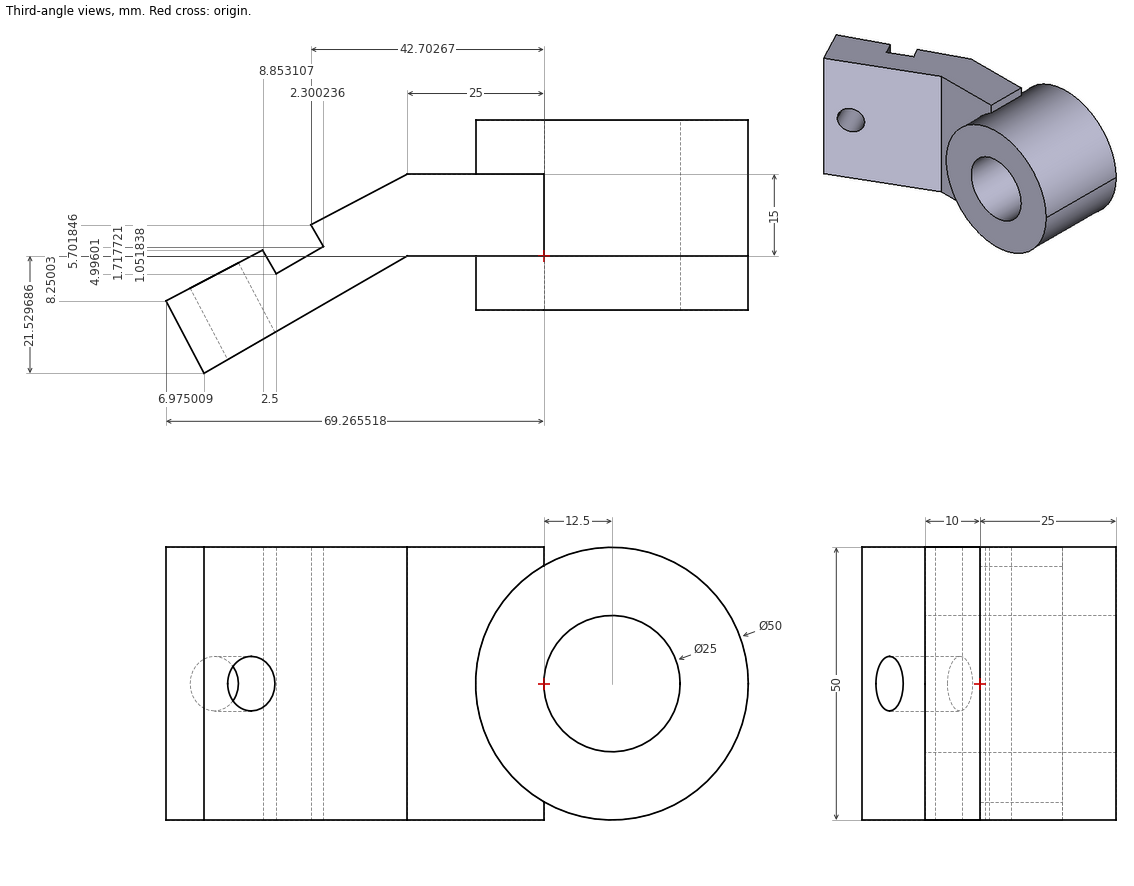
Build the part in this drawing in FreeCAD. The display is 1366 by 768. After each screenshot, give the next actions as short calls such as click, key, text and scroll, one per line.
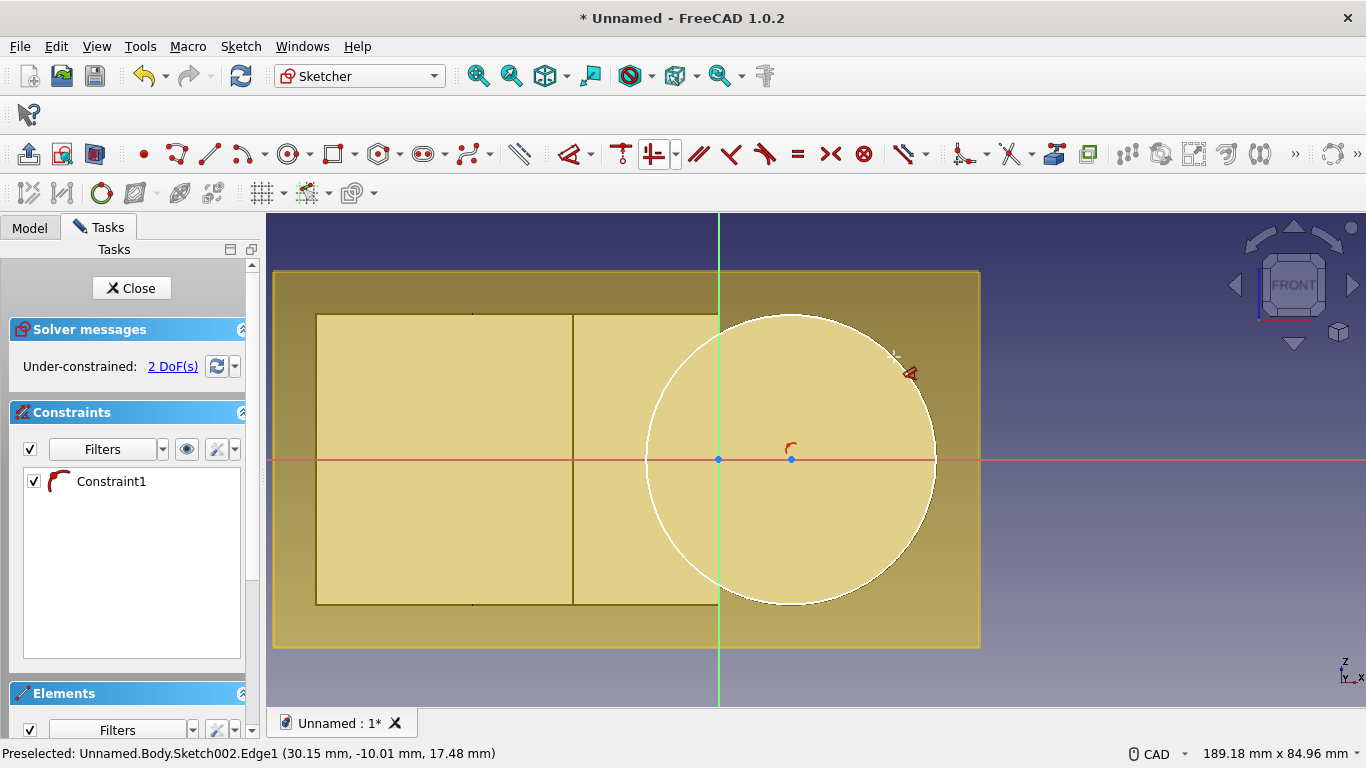
click(893, 357)
click(916, 334)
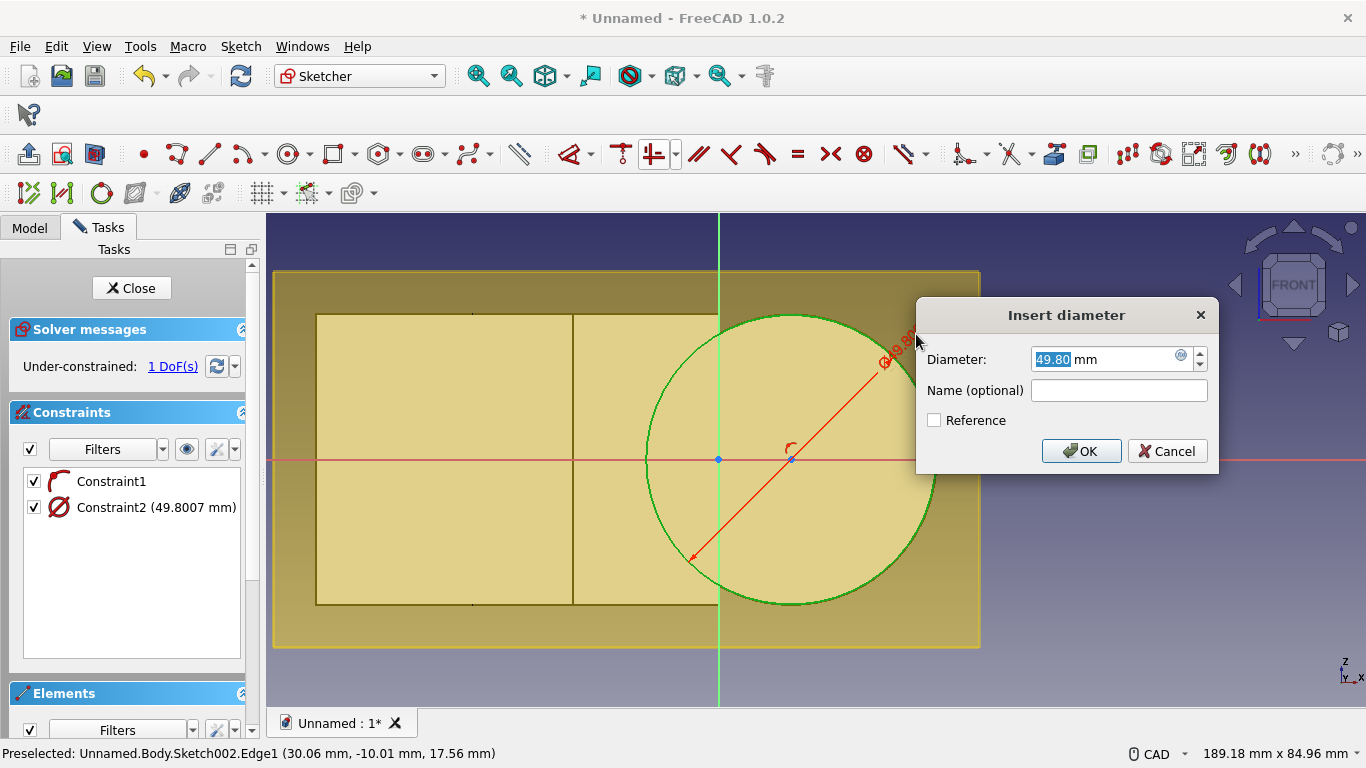
text(50)
key(Return)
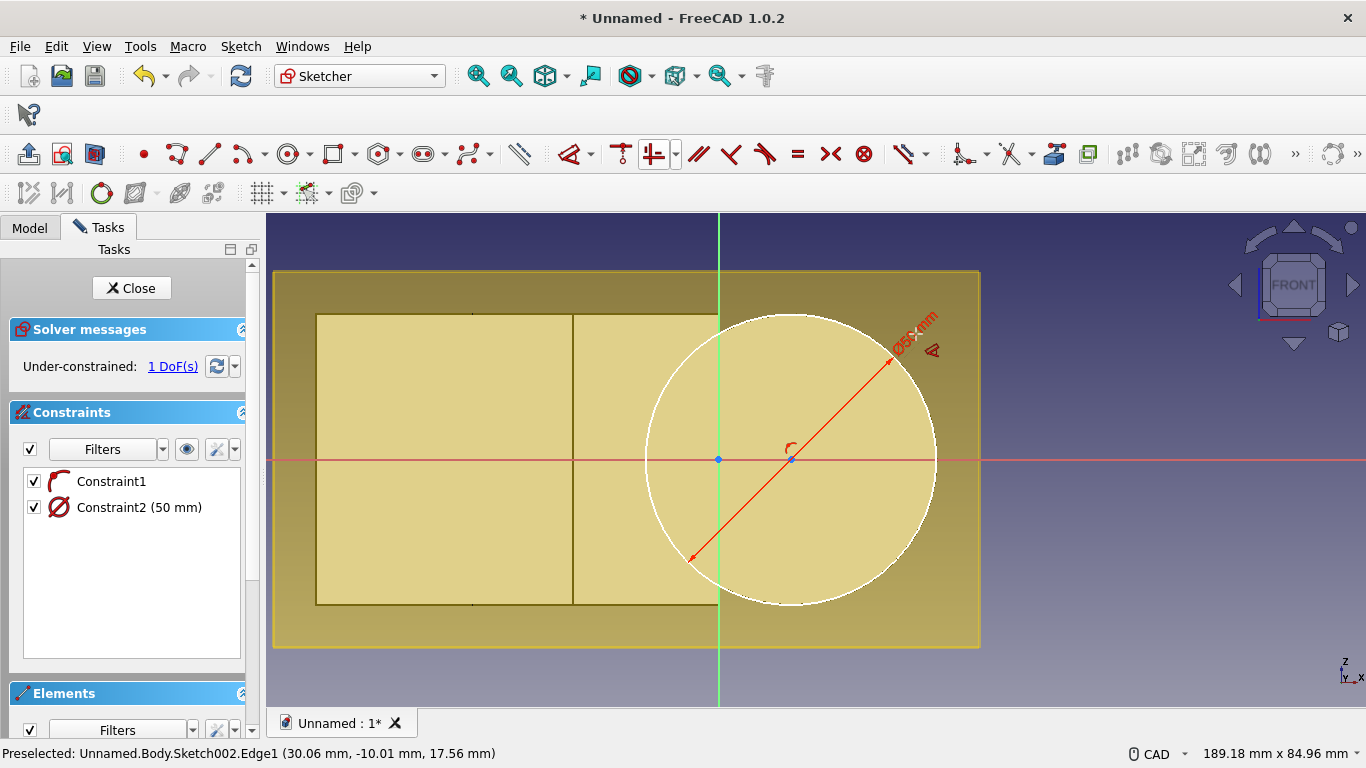
click(791, 460)
click(755, 494)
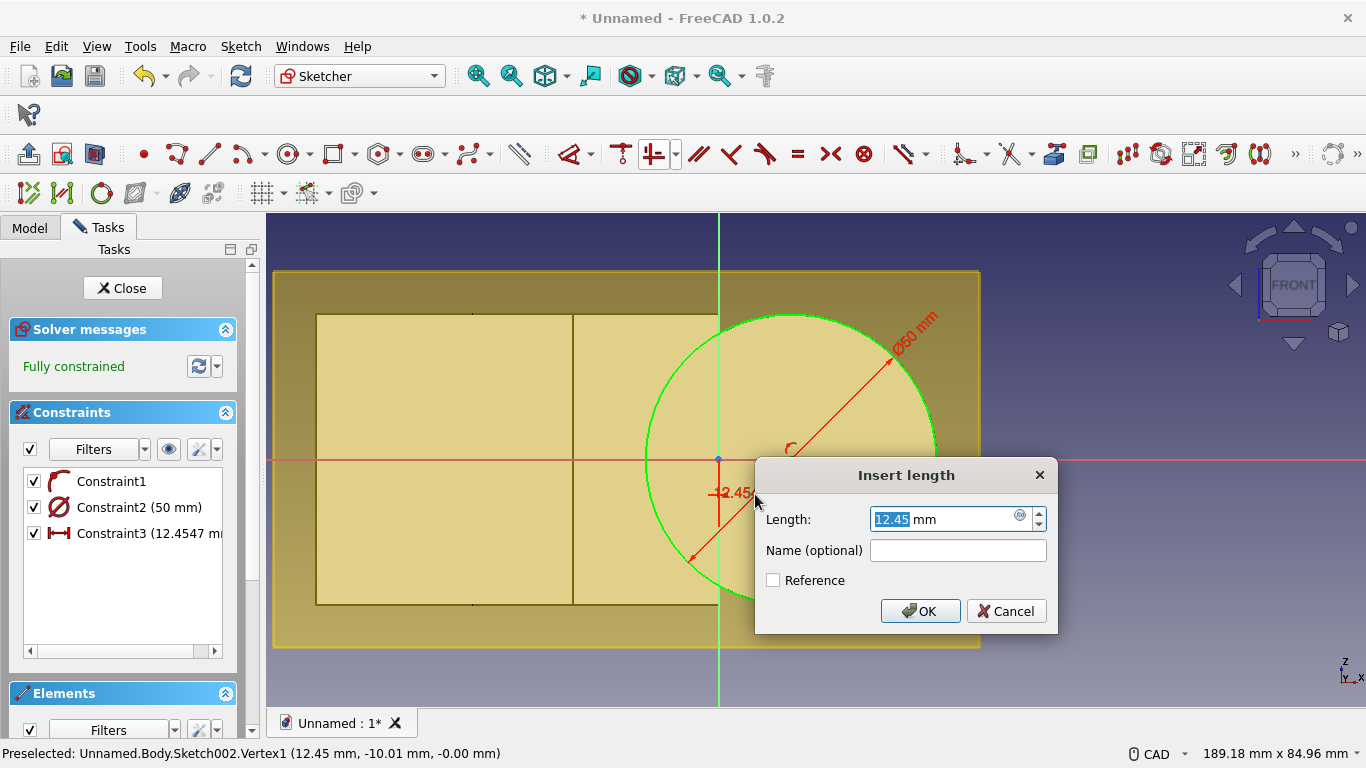
text(12.5)
key(Return)
key(Escape)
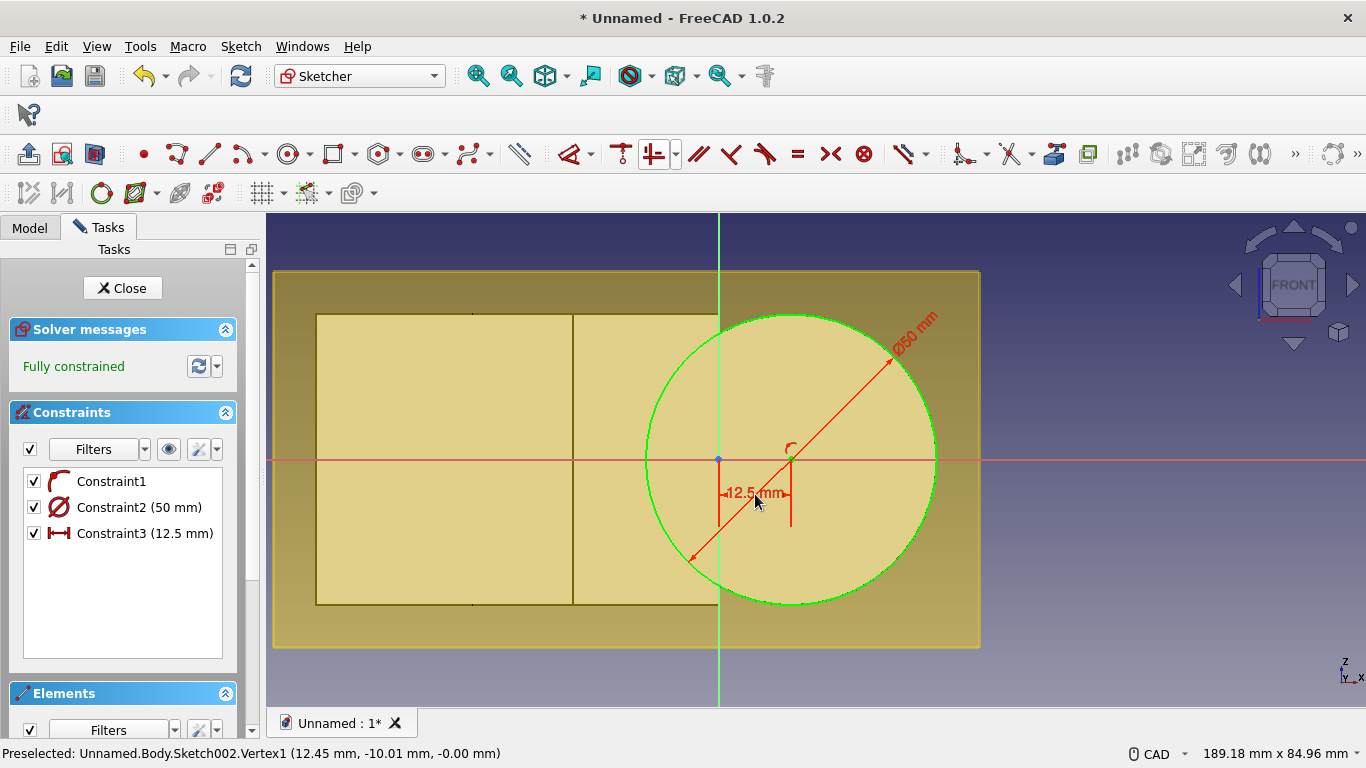
click(123, 288)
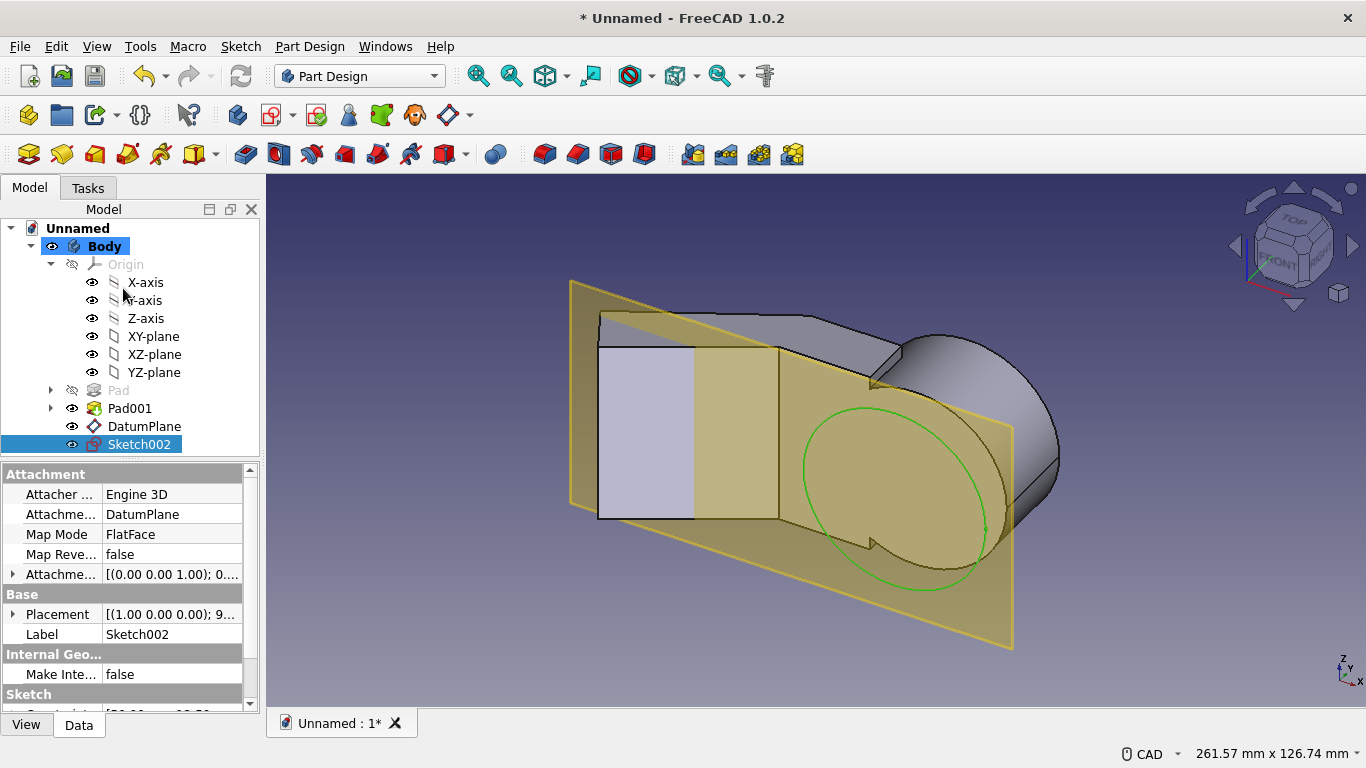
click(29, 154)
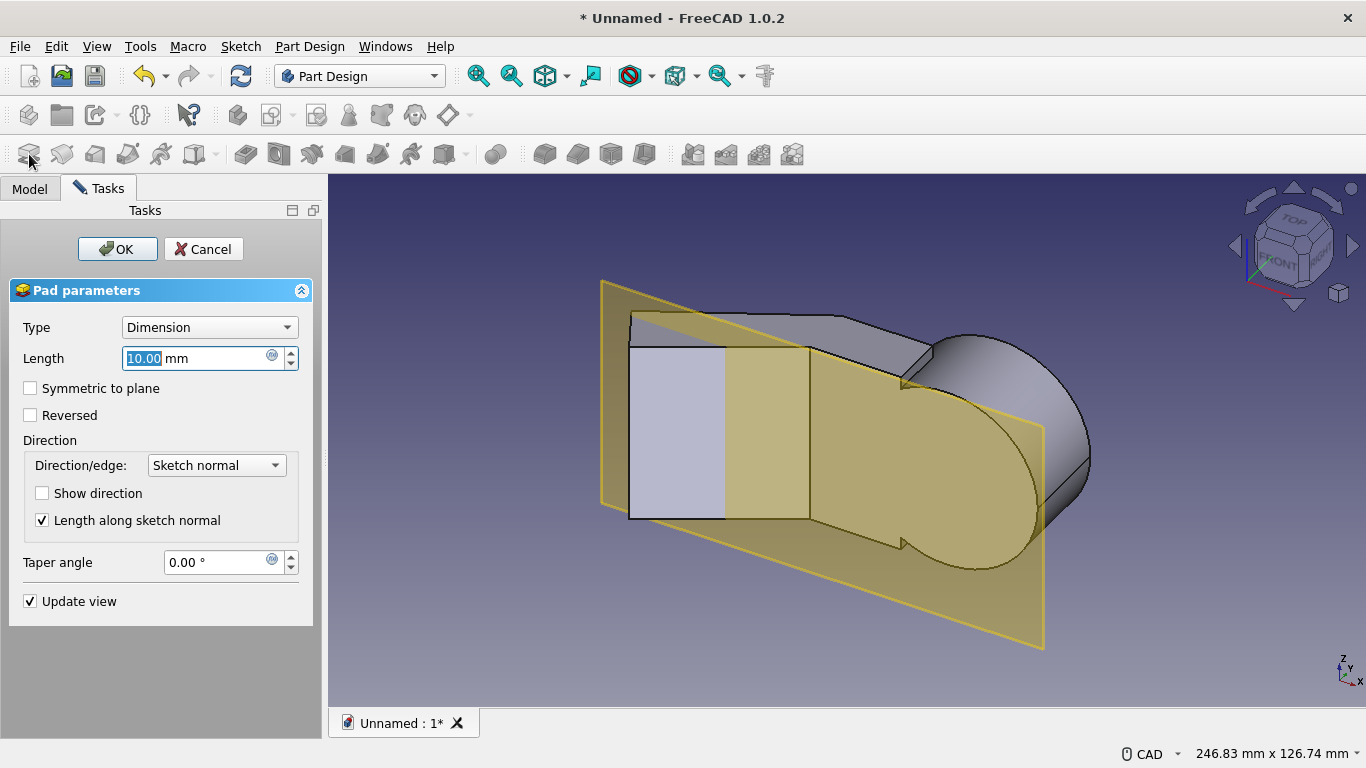
text(10)
key(Tab)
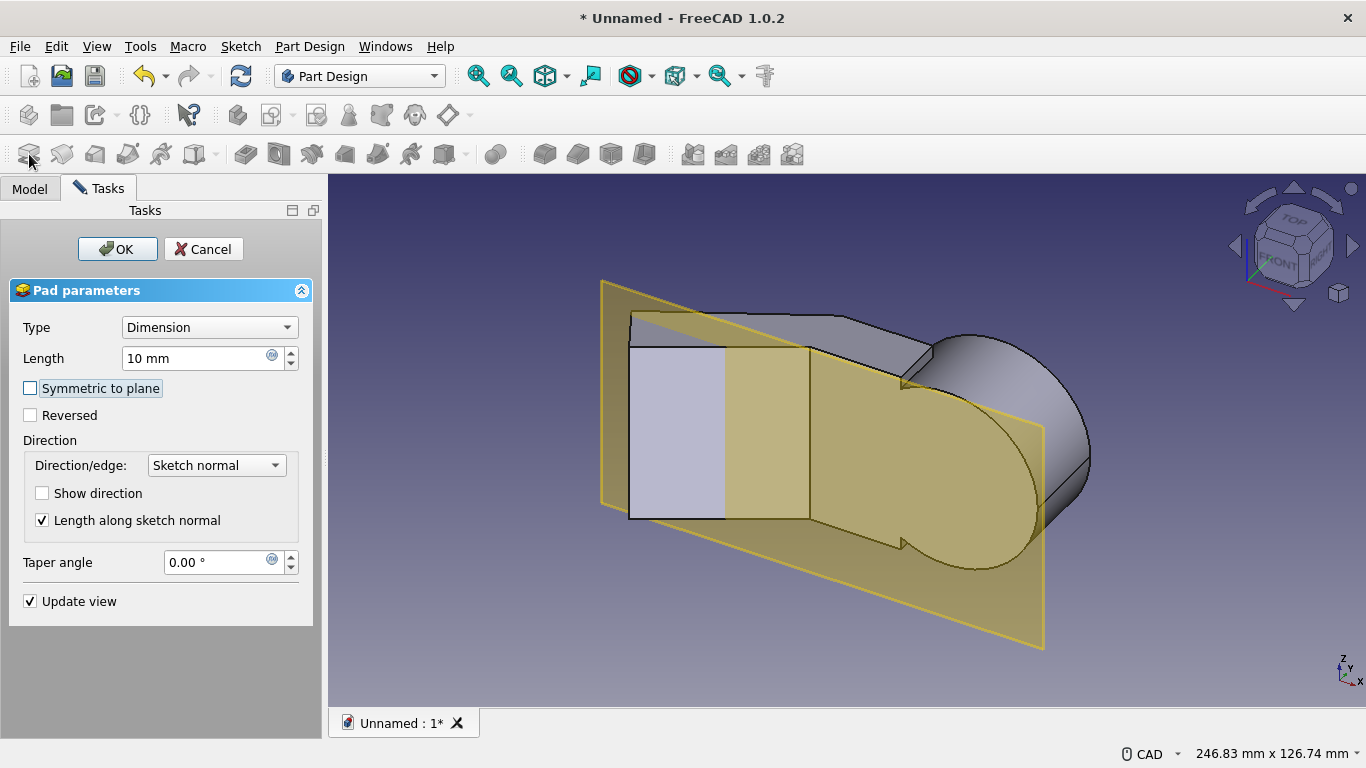
click(31, 415)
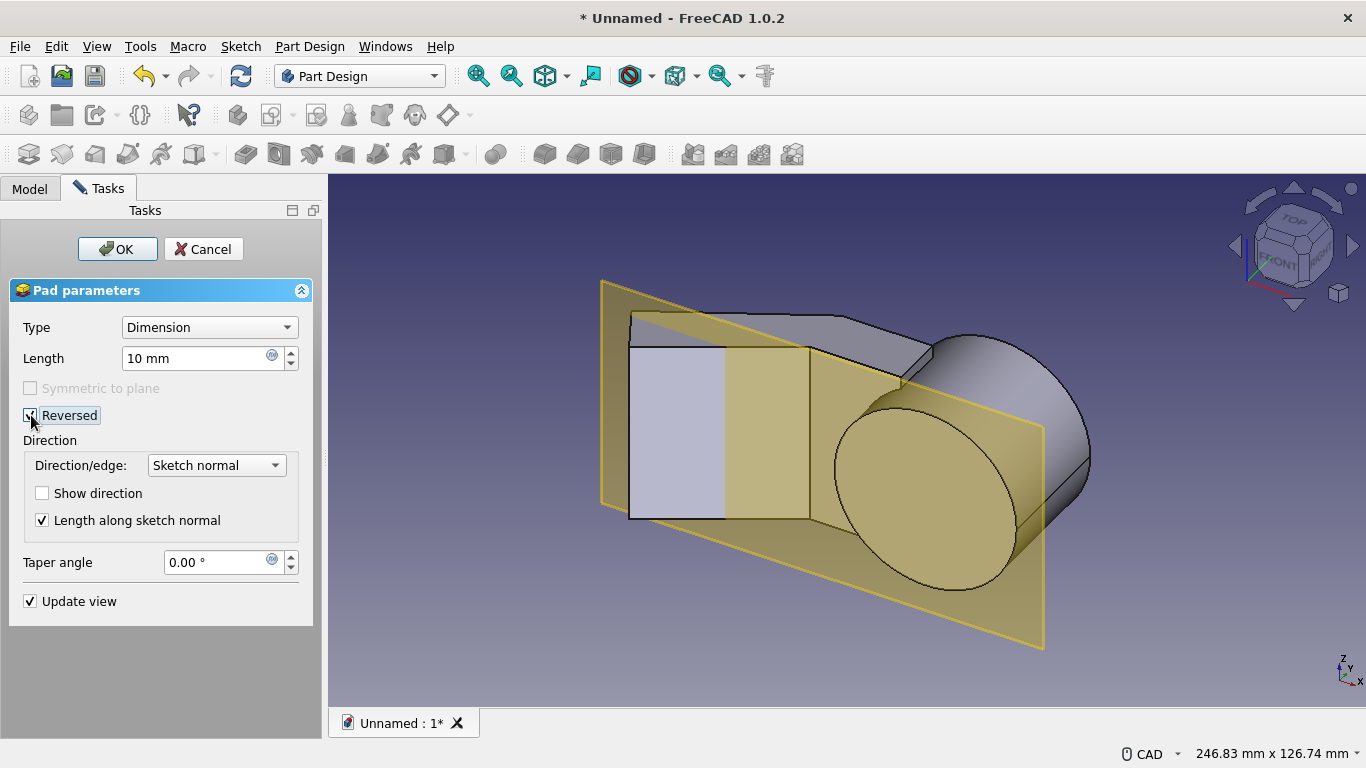
click(118, 249)